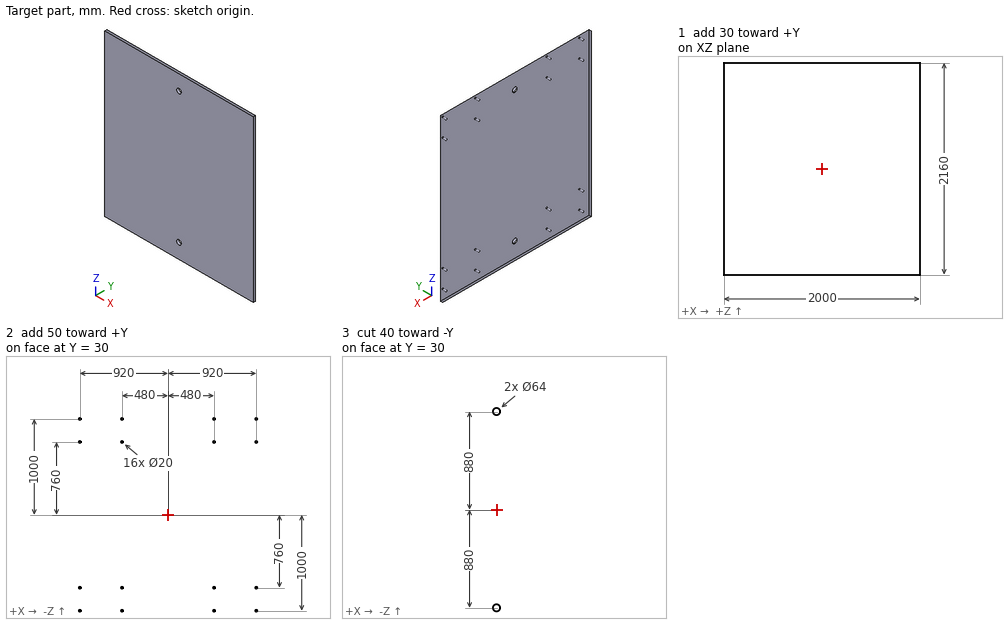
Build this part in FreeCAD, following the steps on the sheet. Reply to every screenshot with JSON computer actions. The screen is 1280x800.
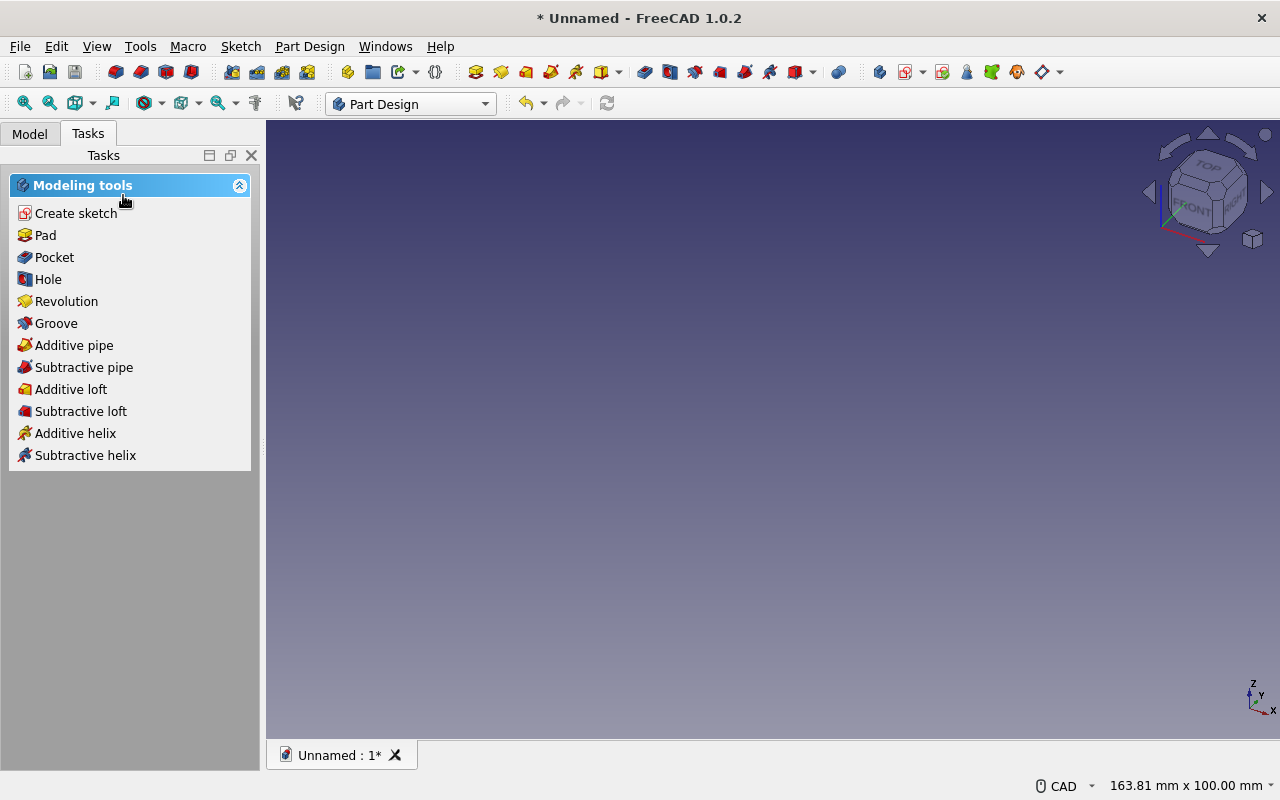
{"action": "left_click", "coordinate": [476, 72]}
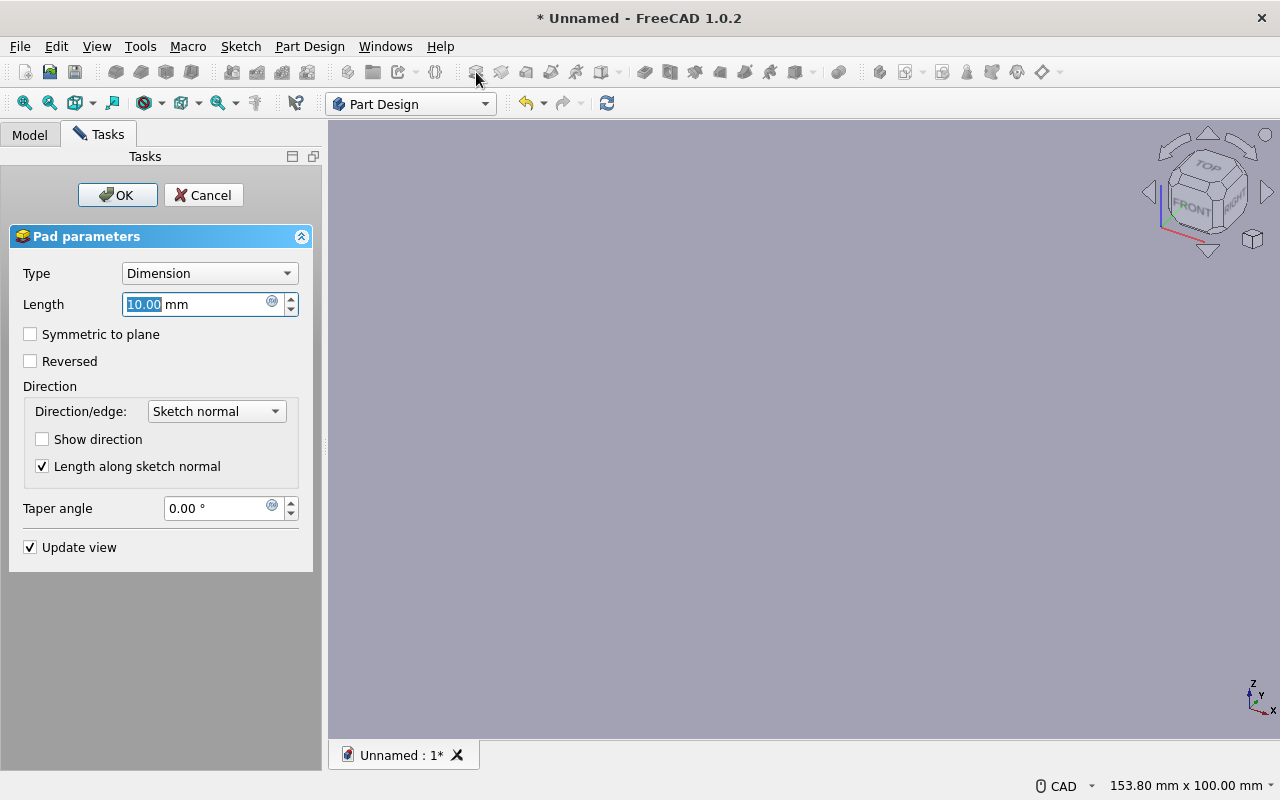
{"action": "type", "text": "30"}
{"action": "key", "text": "Tab"}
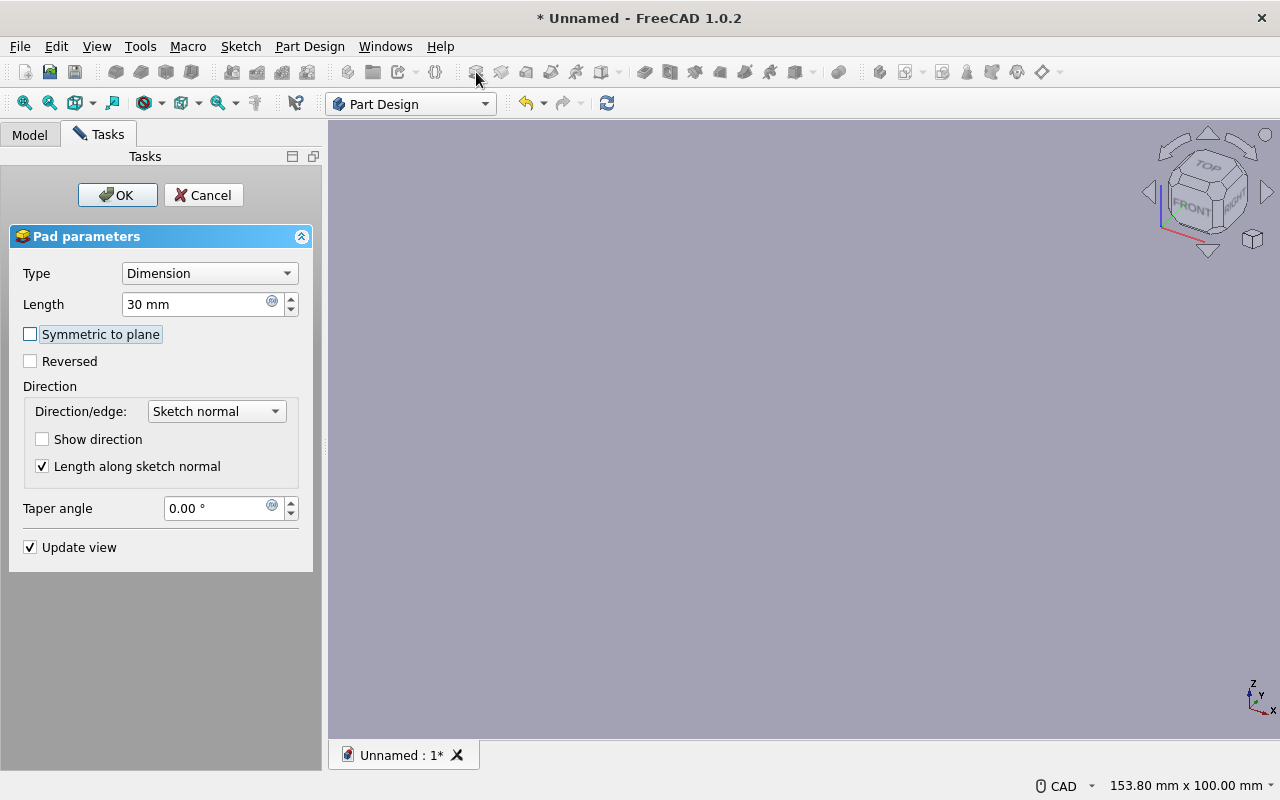
{"action": "left_click", "coordinate": [31, 361]}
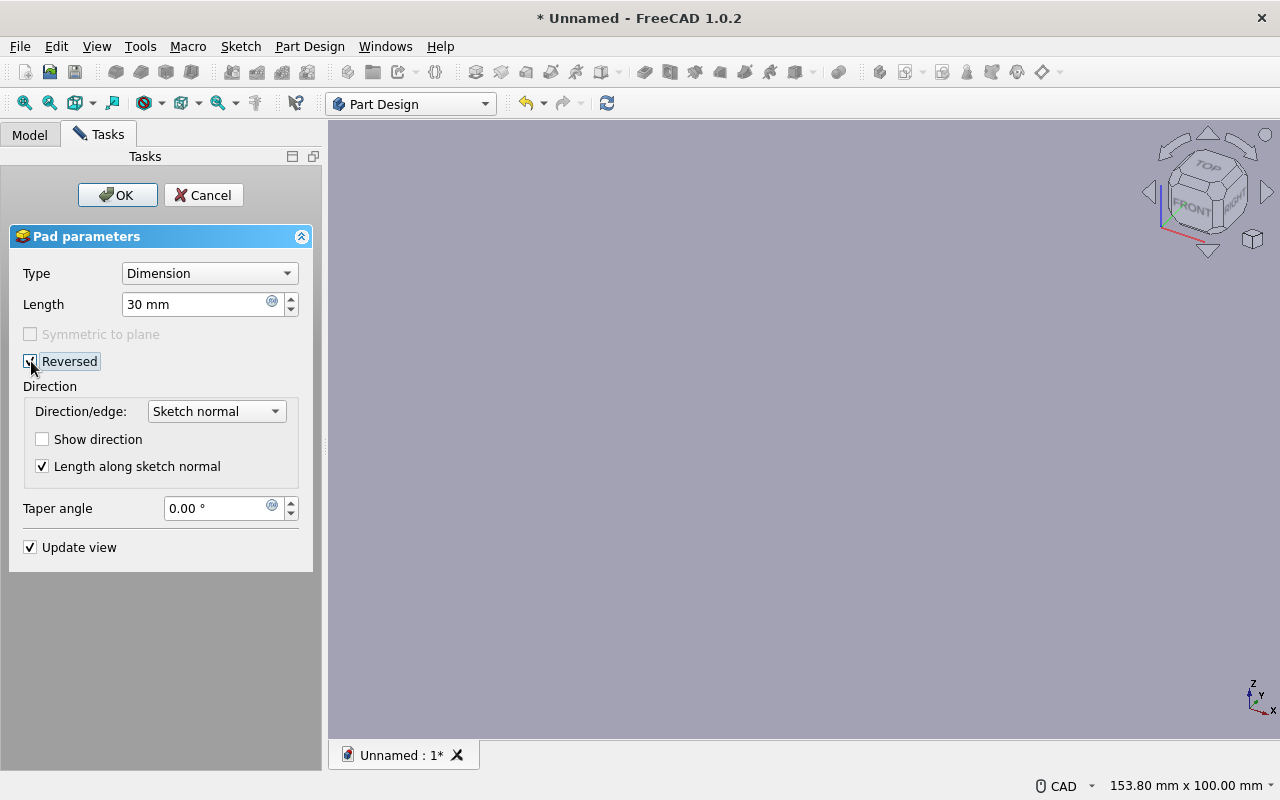
{"action": "left_click", "coordinate": [118, 195]}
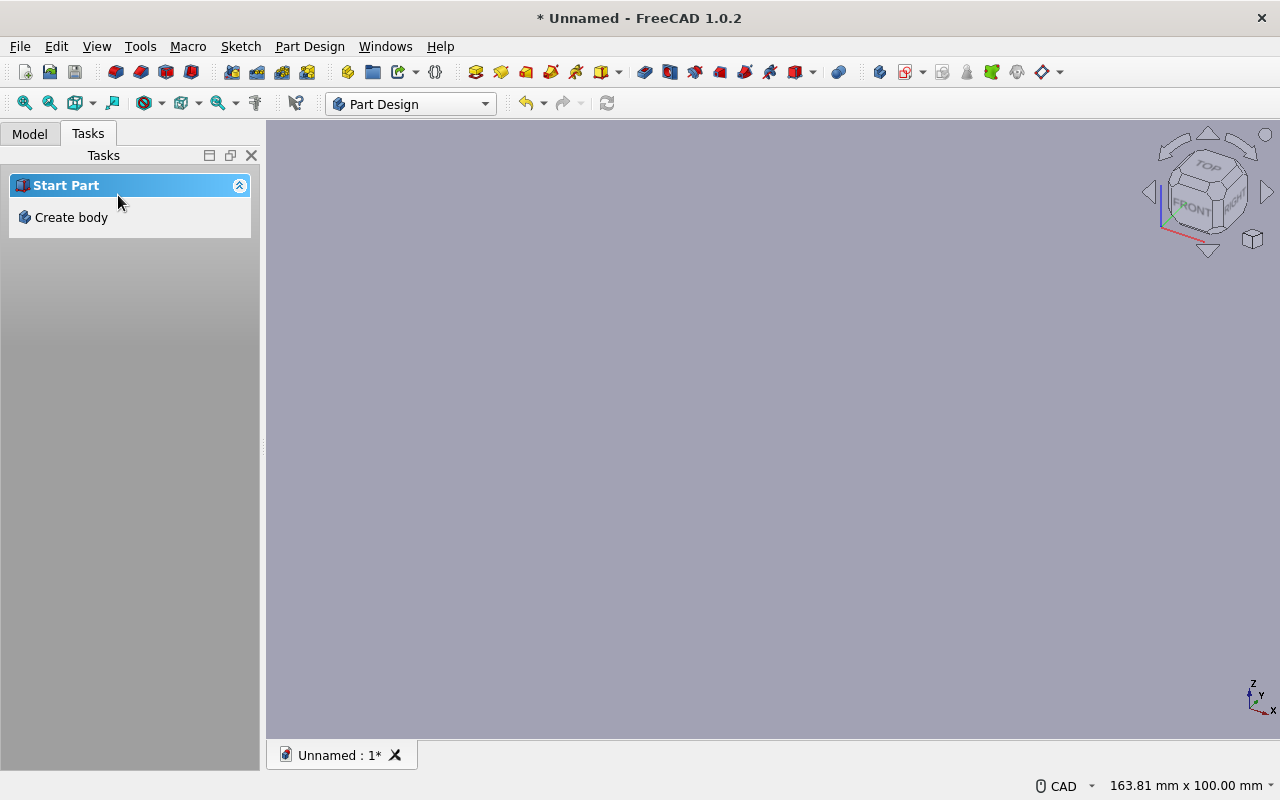
{"action": "left_click", "coordinate": [25, 104]}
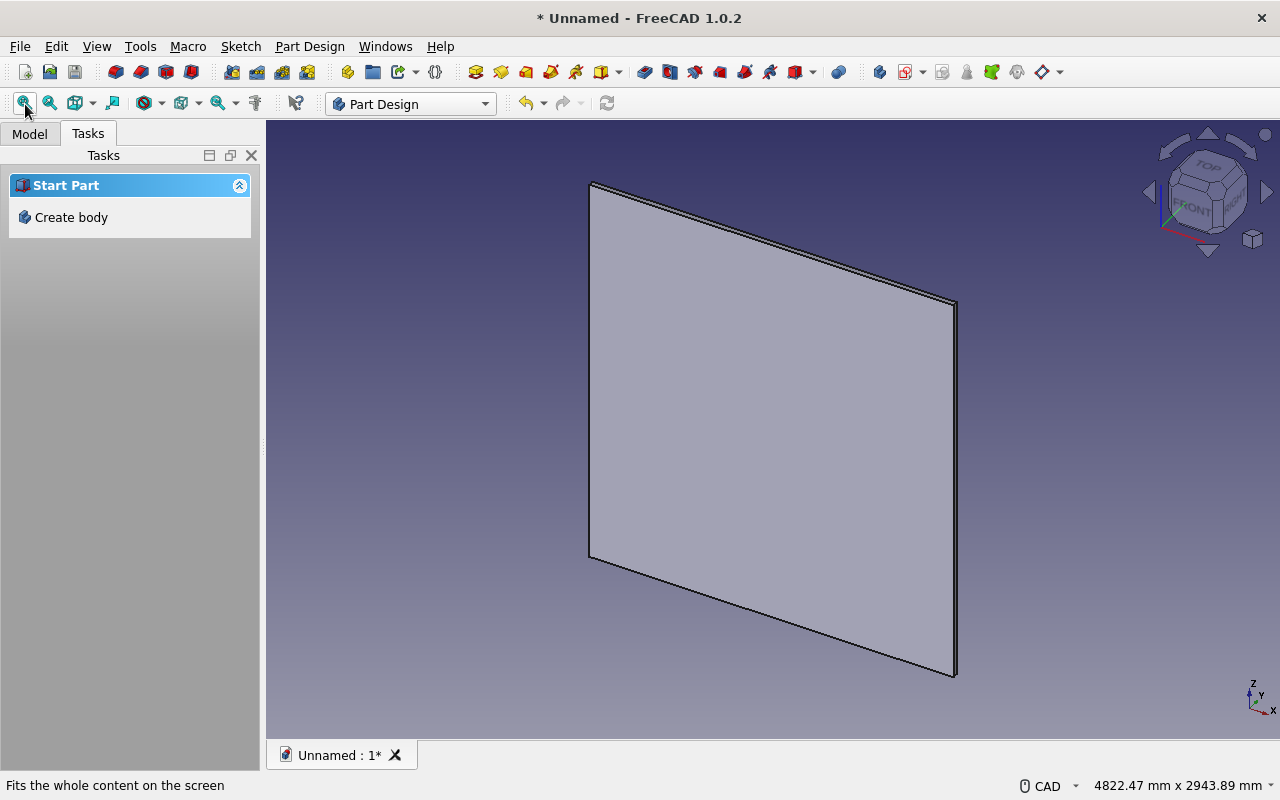
{"action": "key", "text": "4"}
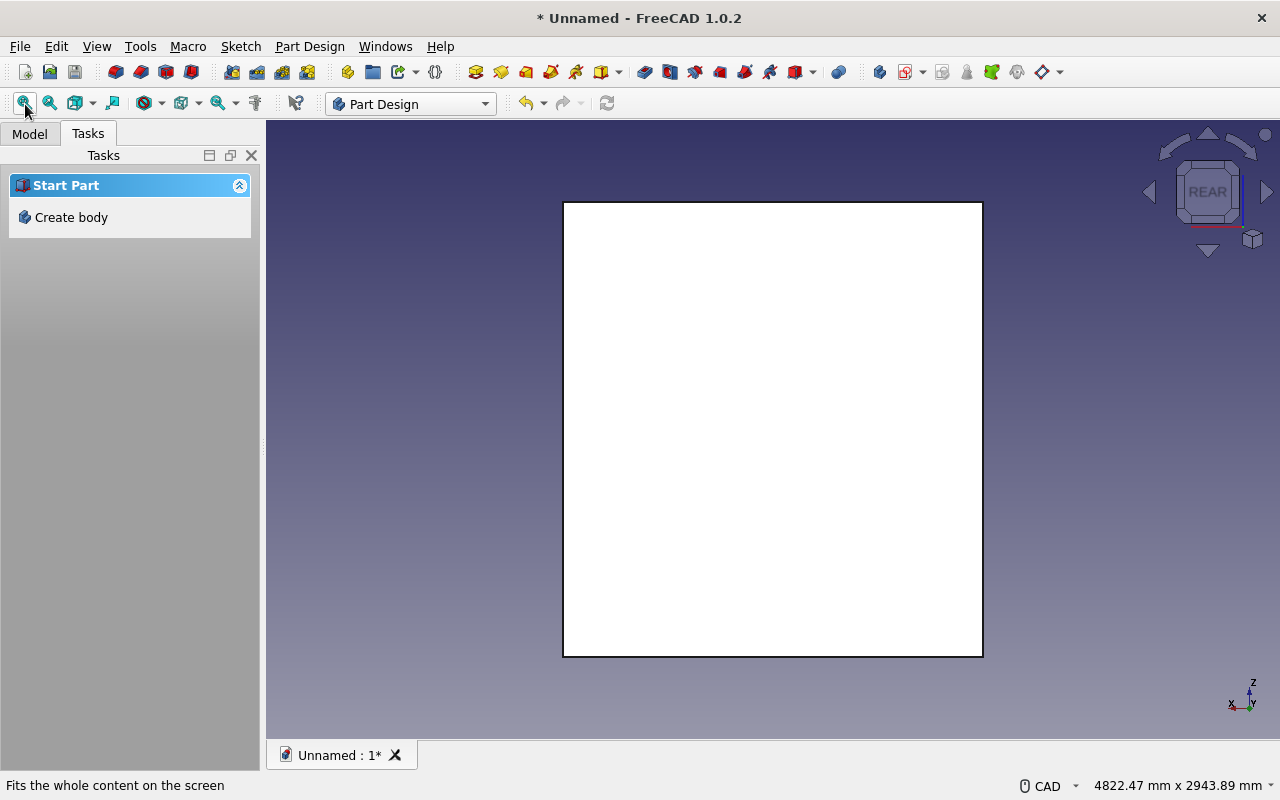
{"action": "left_click", "coordinate": [773, 429]}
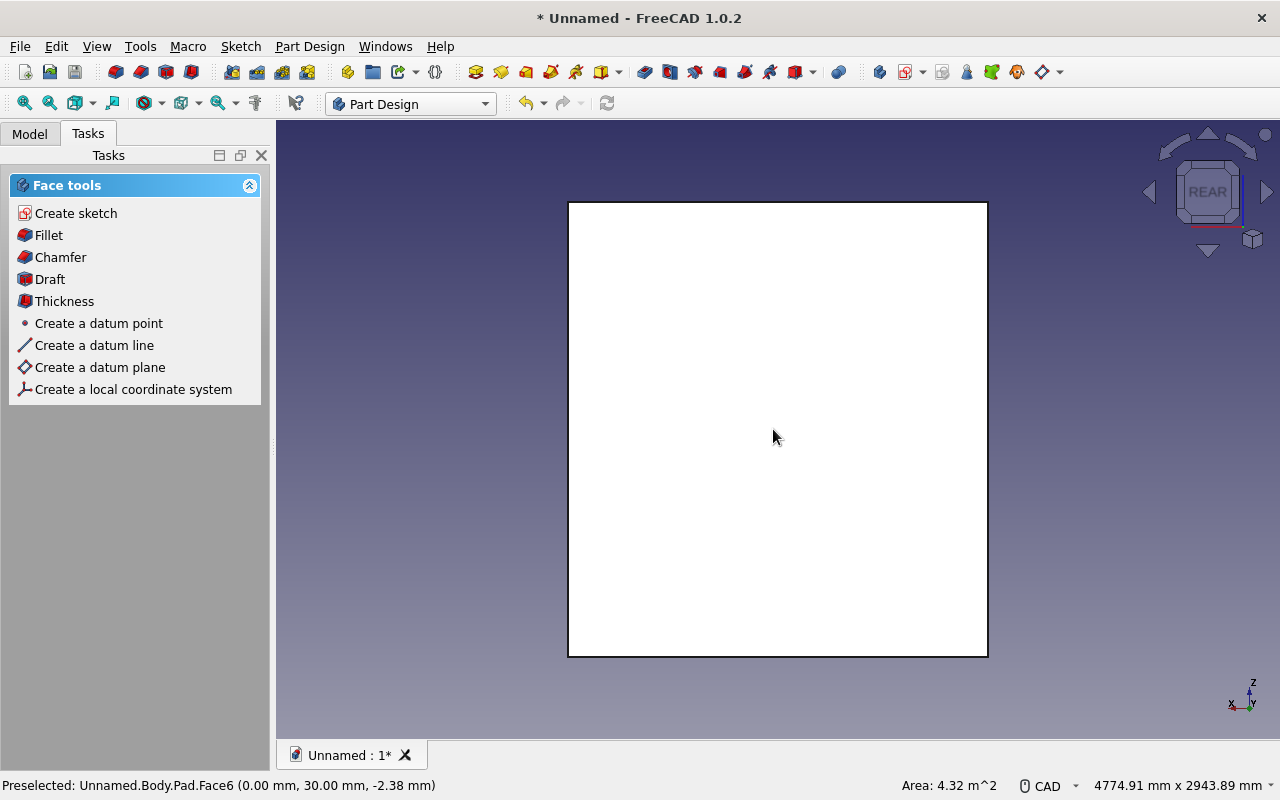
{"action": "left_click", "coordinate": [904, 72]}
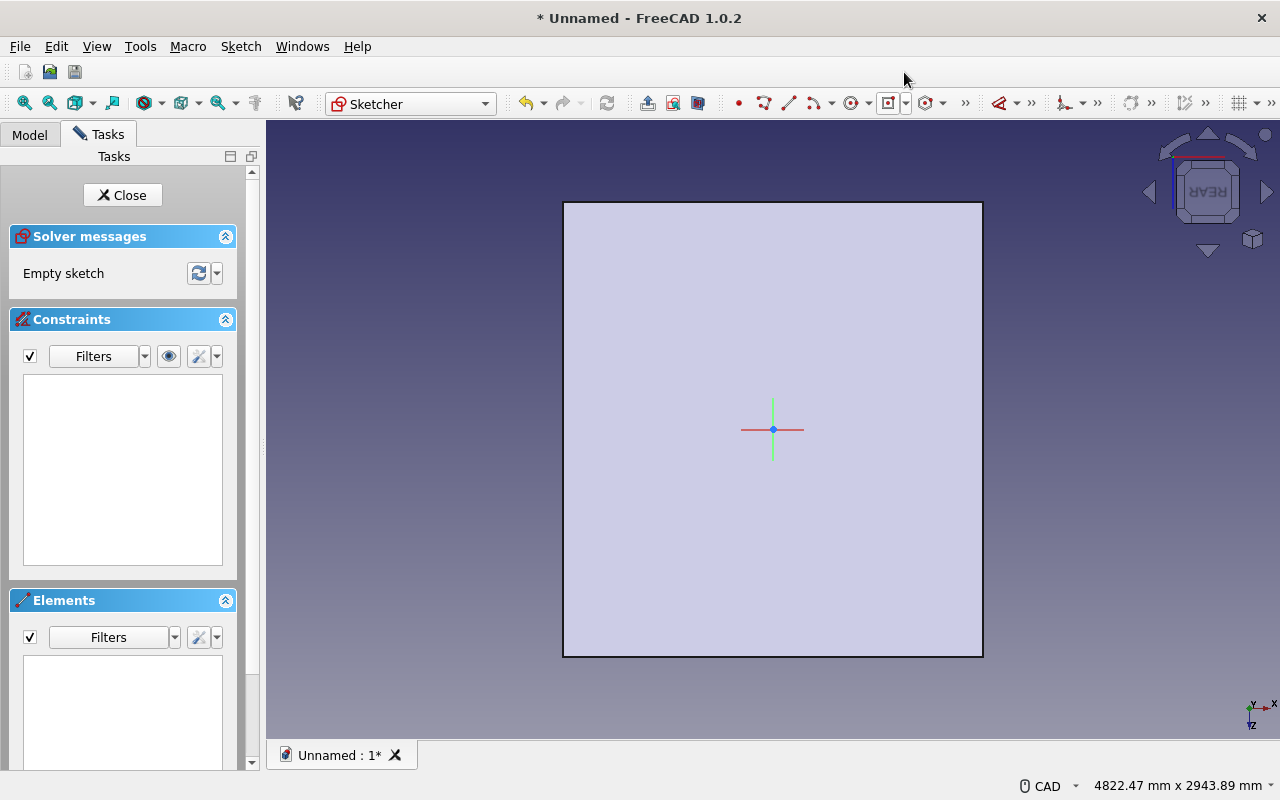
{"action": "left_click", "coordinate": [850, 104]}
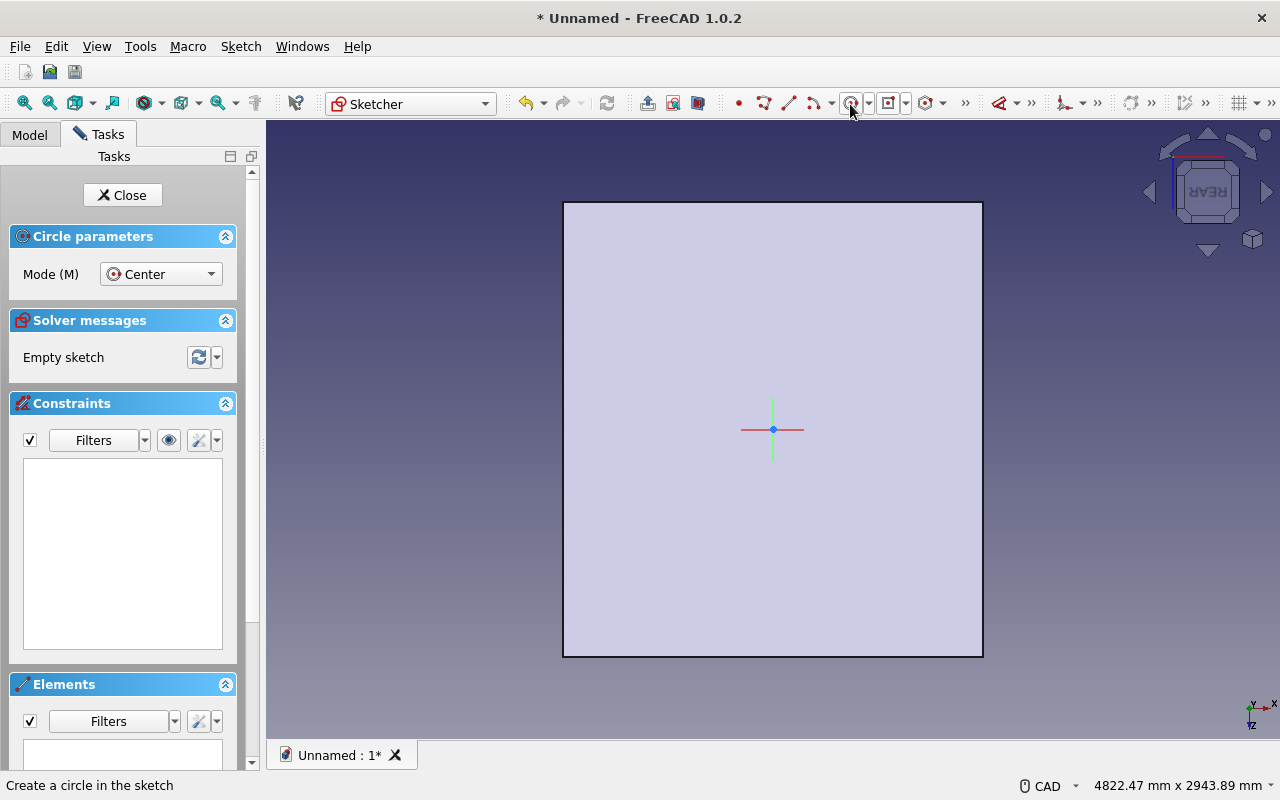
{"action": "scroll", "coordinate": [580, 219], "scroll_direction": "up", "scroll_amount": 12}